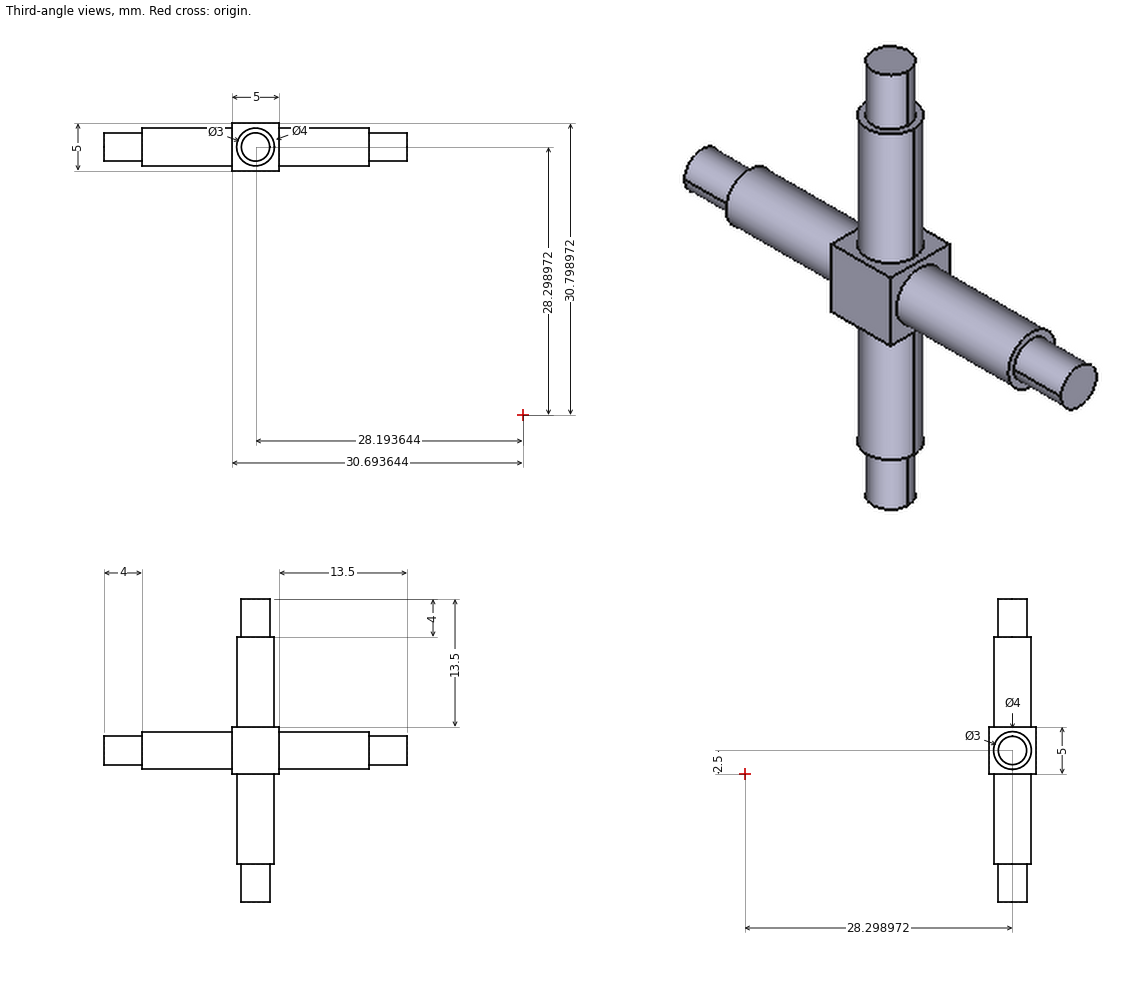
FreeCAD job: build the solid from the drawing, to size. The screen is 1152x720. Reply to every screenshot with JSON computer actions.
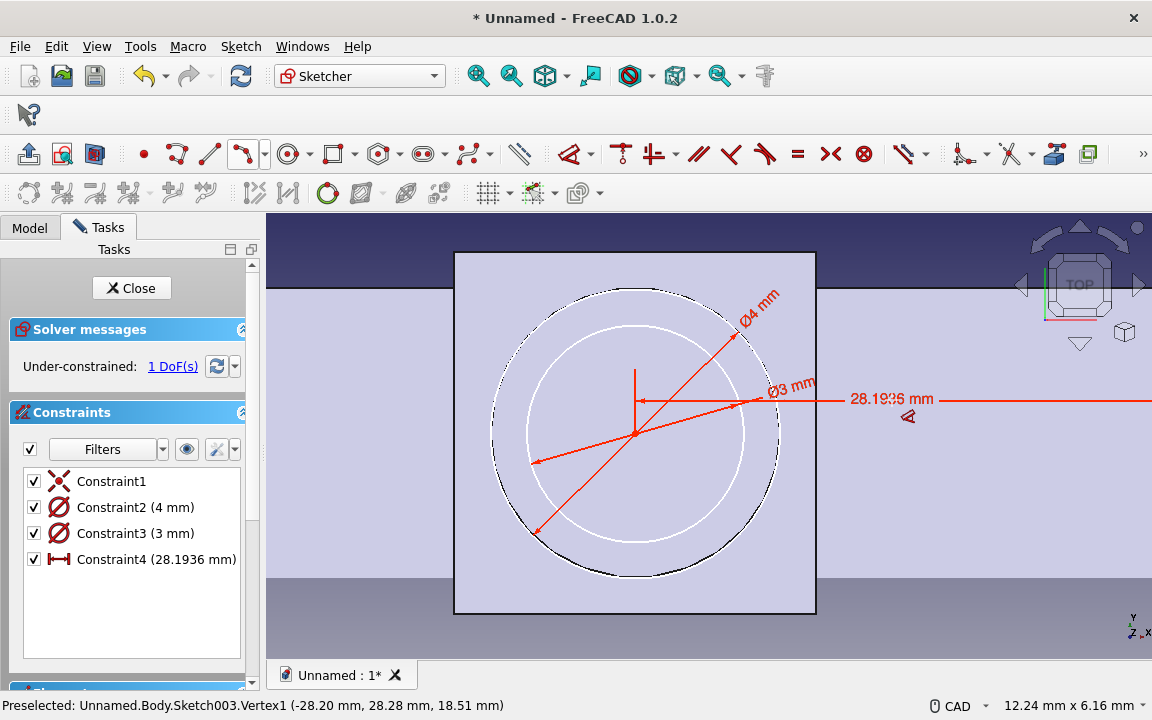
{"action": "left_click", "coordinate": [635, 434]}
{"action": "left_click", "coordinate": [601, 487]}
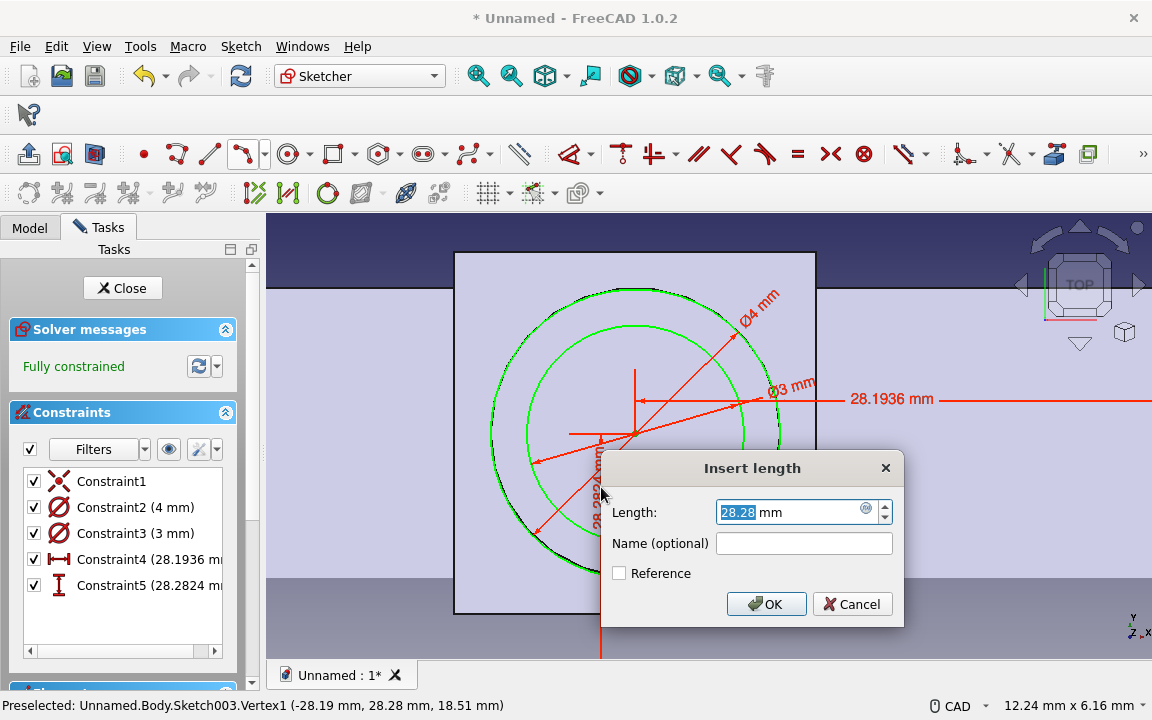
{"action": "type", "text": "28.298972"}
{"action": "key", "text": "Return"}
{"action": "key", "text": "Escape"}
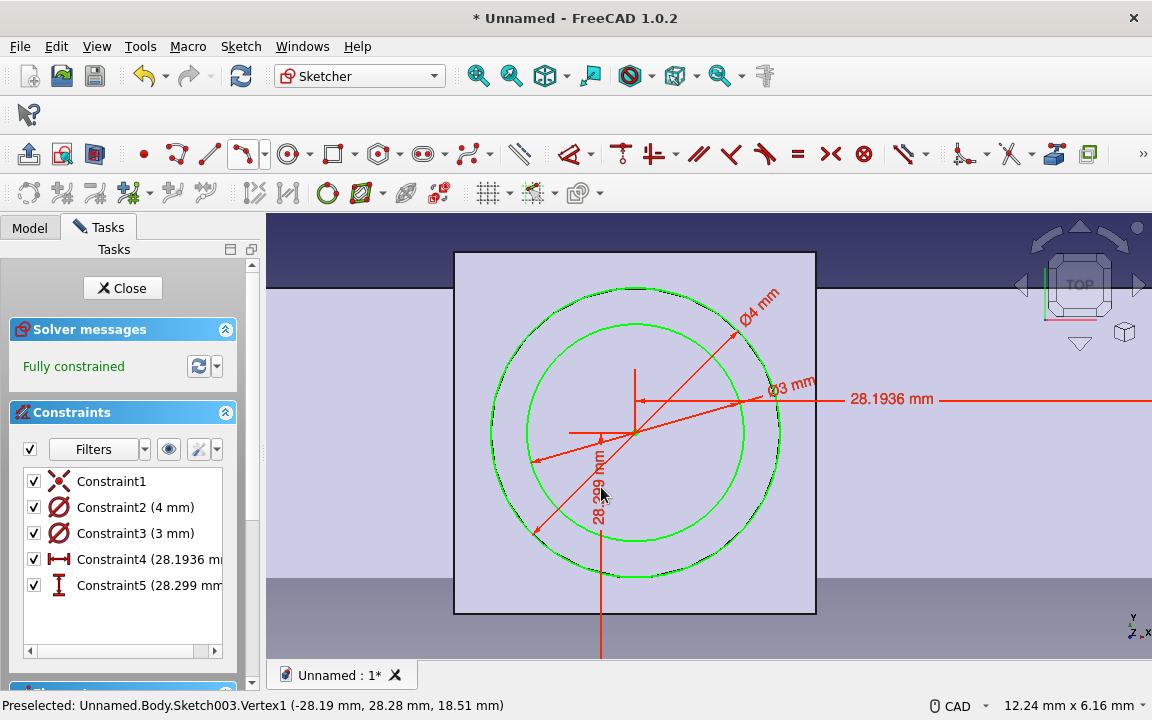
{"action": "left_click", "coordinate": [123, 288]}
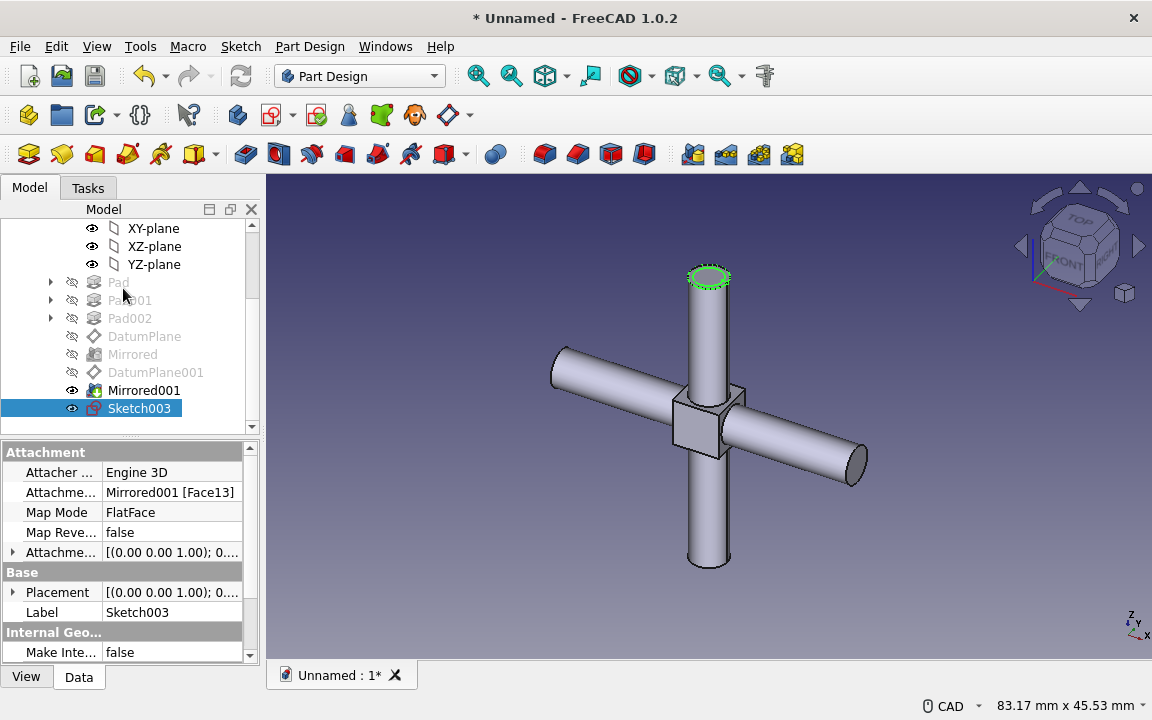
{"action": "left_click", "coordinate": [246, 154]}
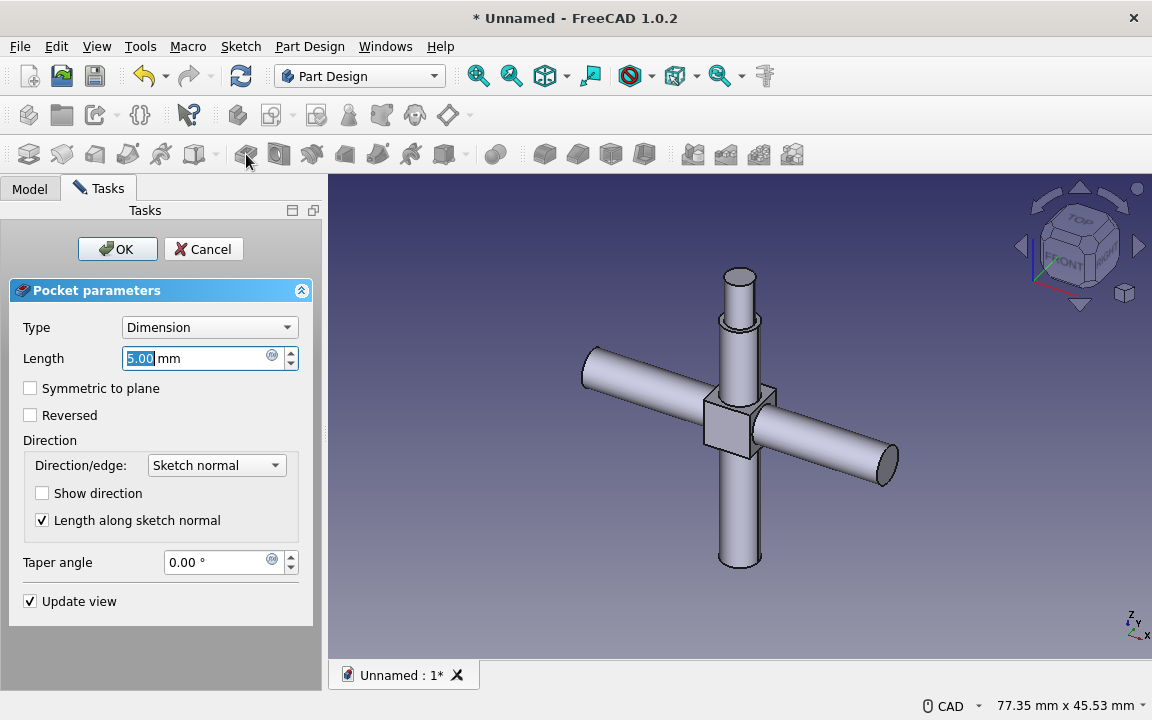
{"action": "type", "text": "4"}
{"action": "key", "text": "Tab"}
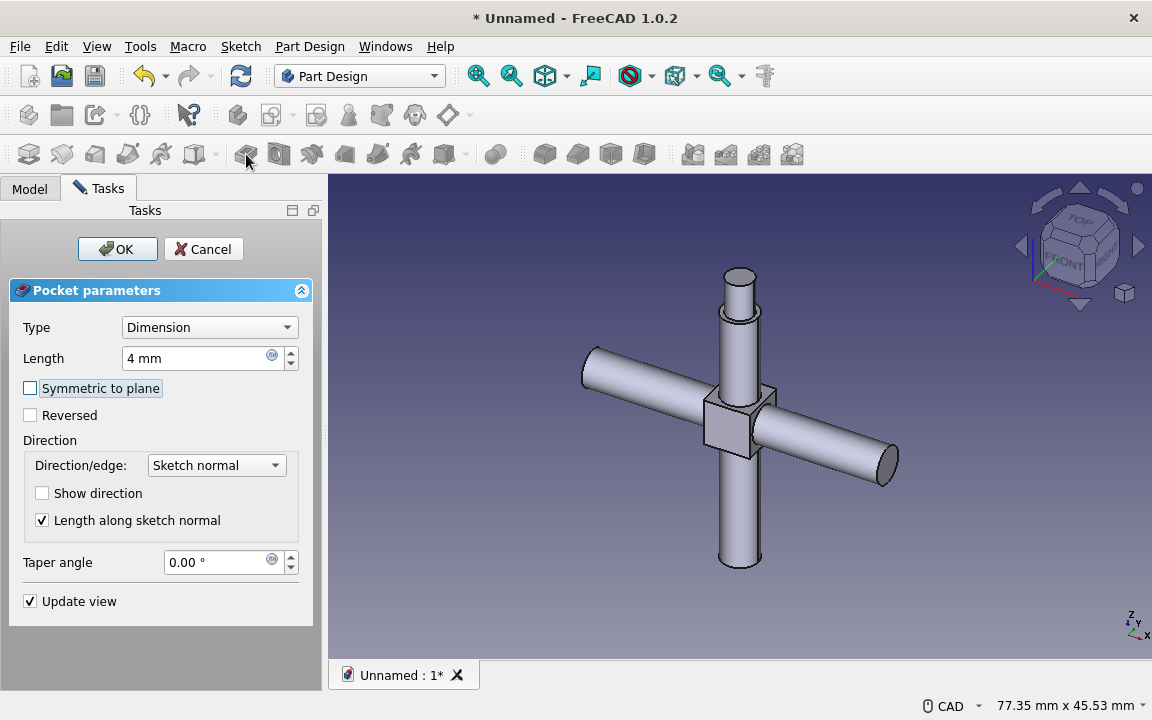
{"action": "left_click", "coordinate": [118, 249]}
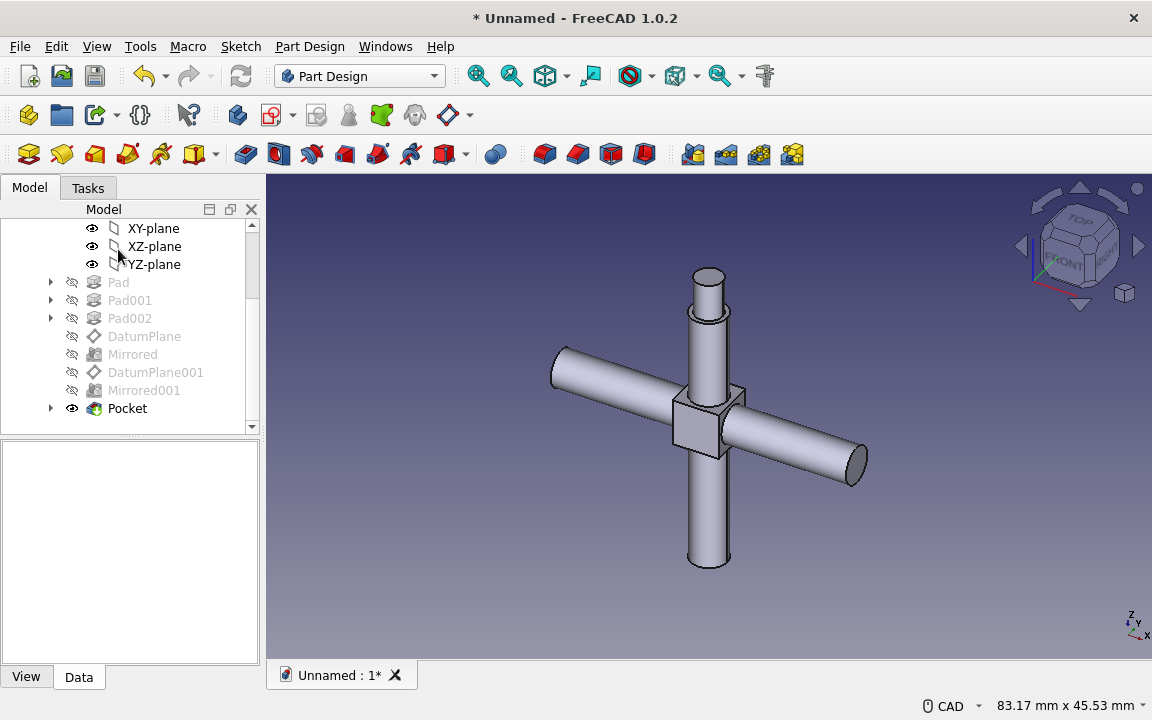
{"action": "scroll", "coordinate": [161, 314], "scroll_direction": "down", "scroll_amount": 3}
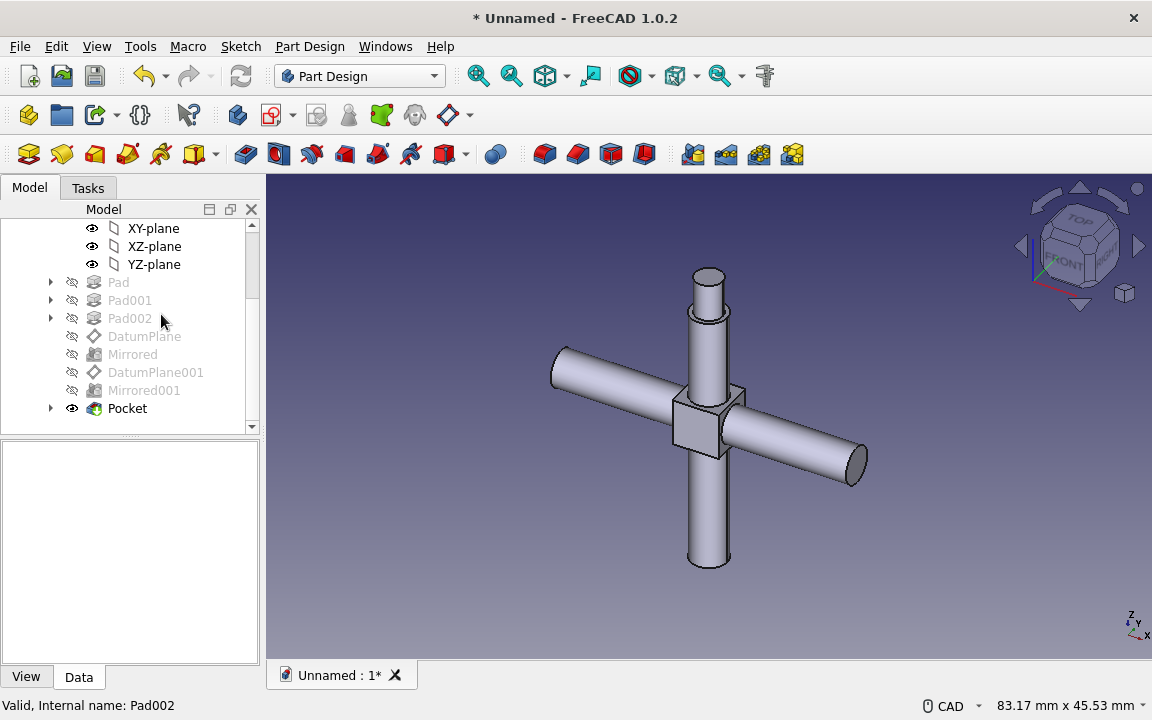
{"action": "scroll", "coordinate": [161, 314], "scroll_direction": "up", "scroll_amount": 15}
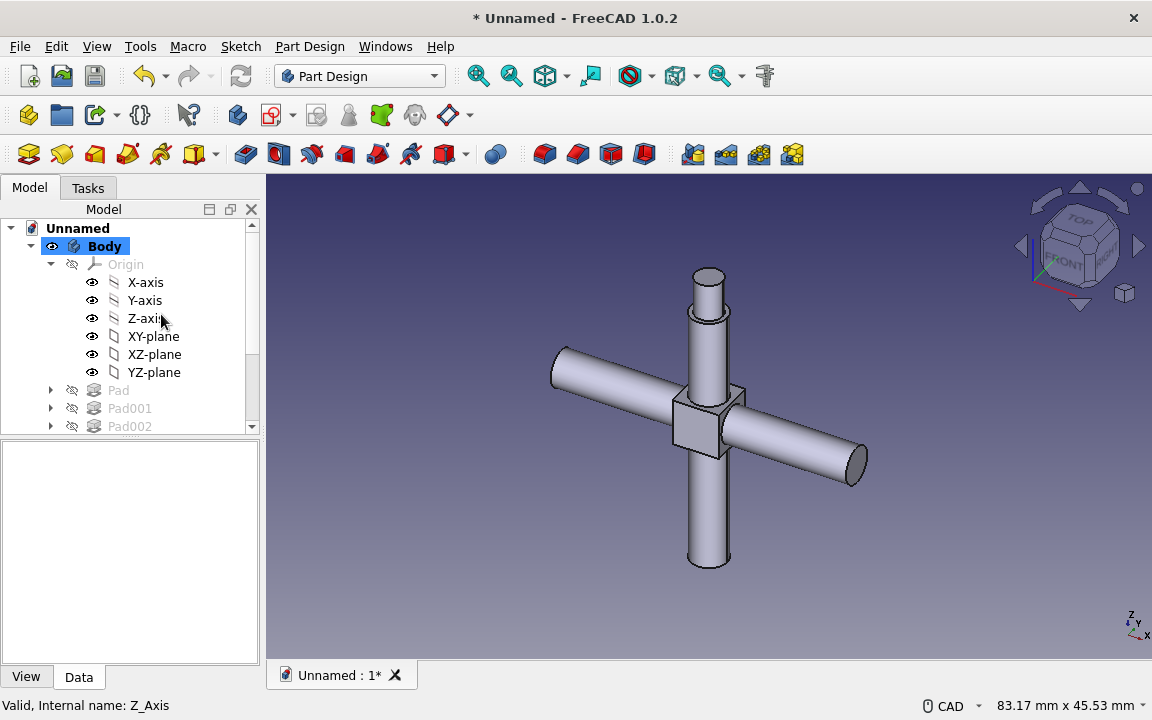
{"action": "left_click", "coordinate": [137, 336]}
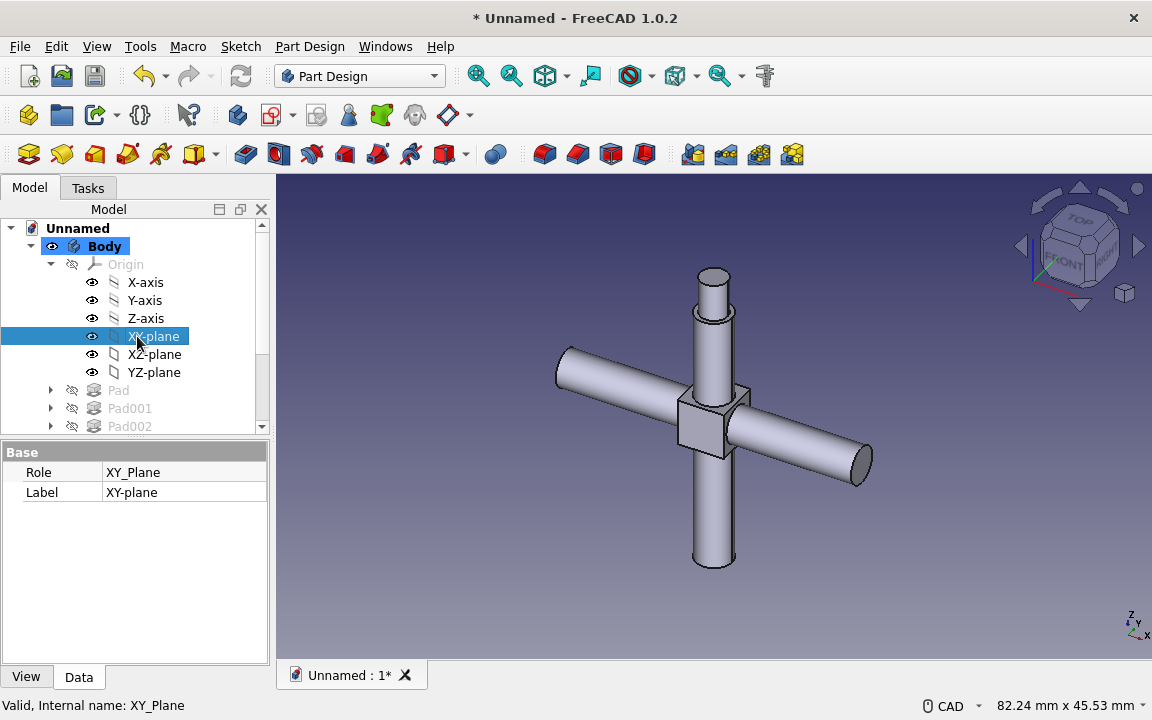
{"action": "left_click", "coordinate": [448, 116]}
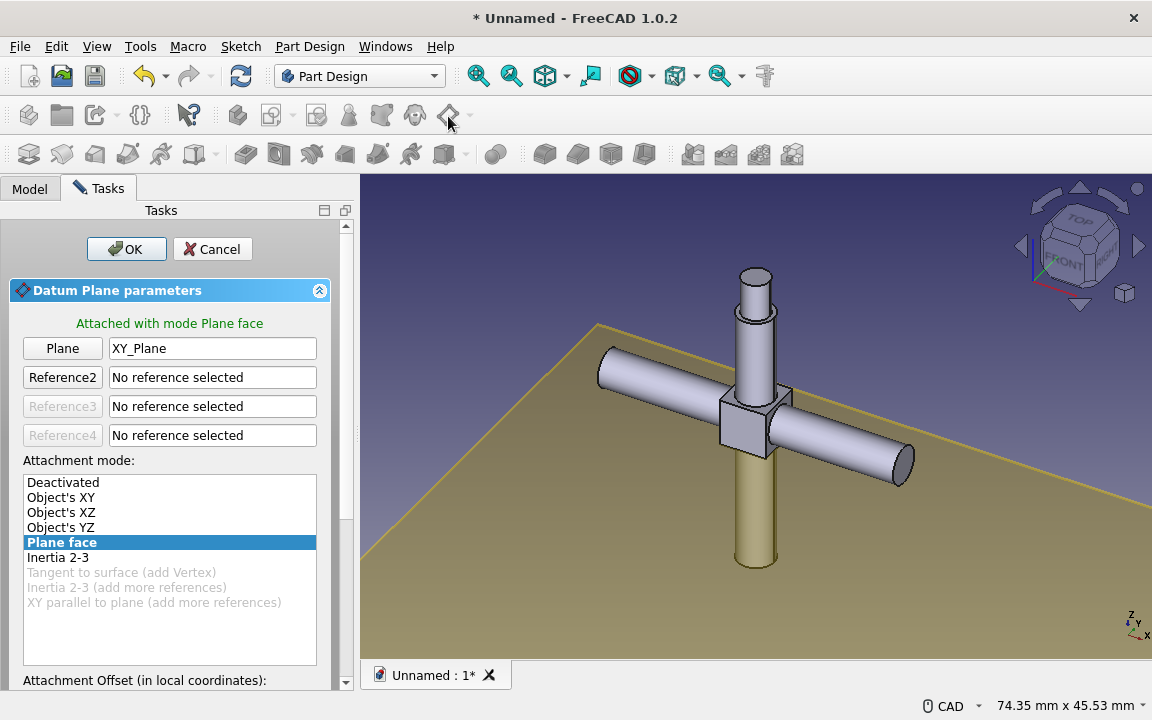
{"action": "scroll", "coordinate": [346, 455], "scroll_direction": "down", "scroll_amount": 3}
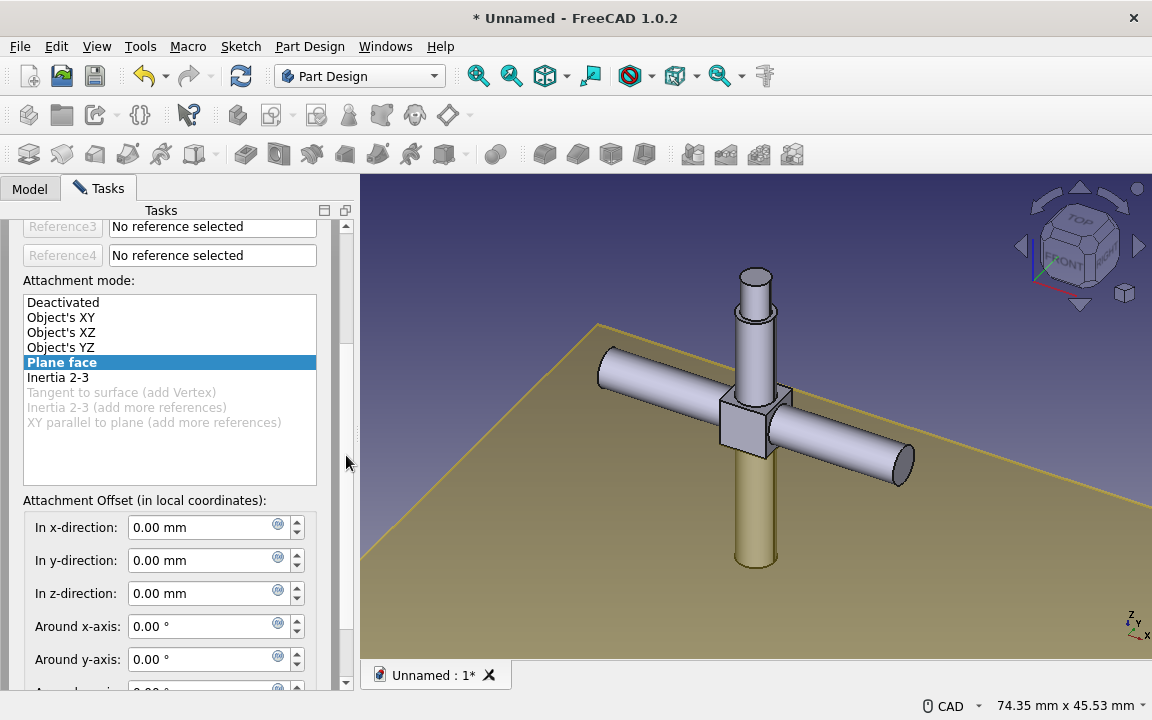
{"action": "triple_click", "coordinate": [210, 594]}